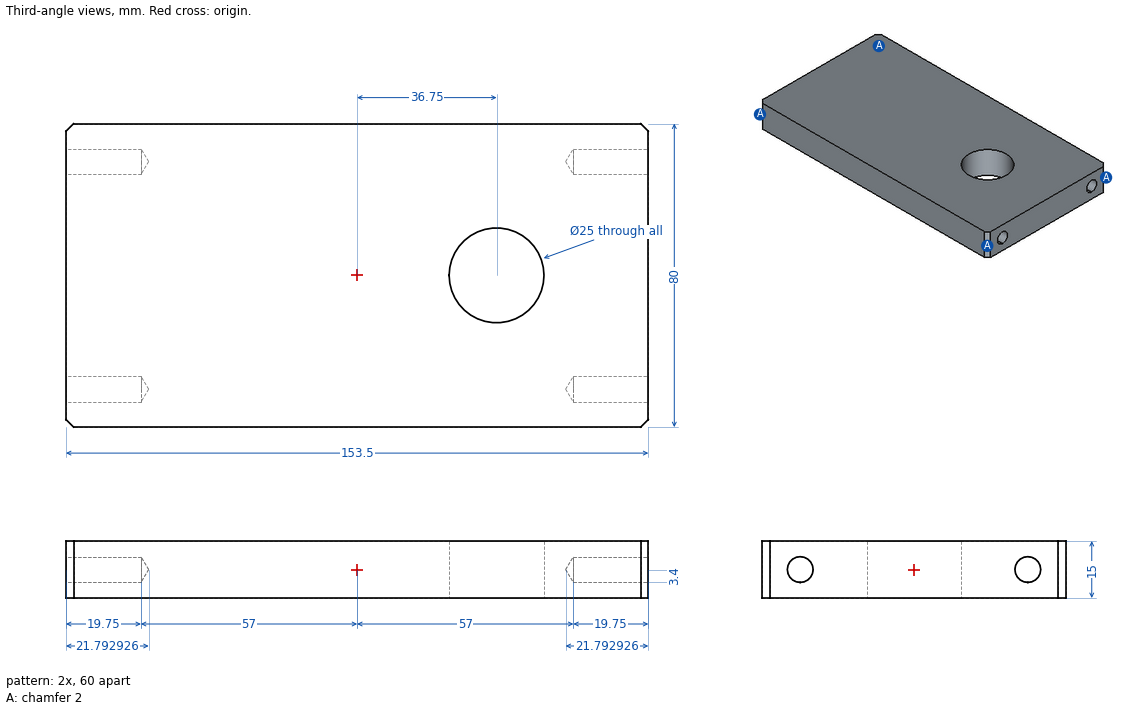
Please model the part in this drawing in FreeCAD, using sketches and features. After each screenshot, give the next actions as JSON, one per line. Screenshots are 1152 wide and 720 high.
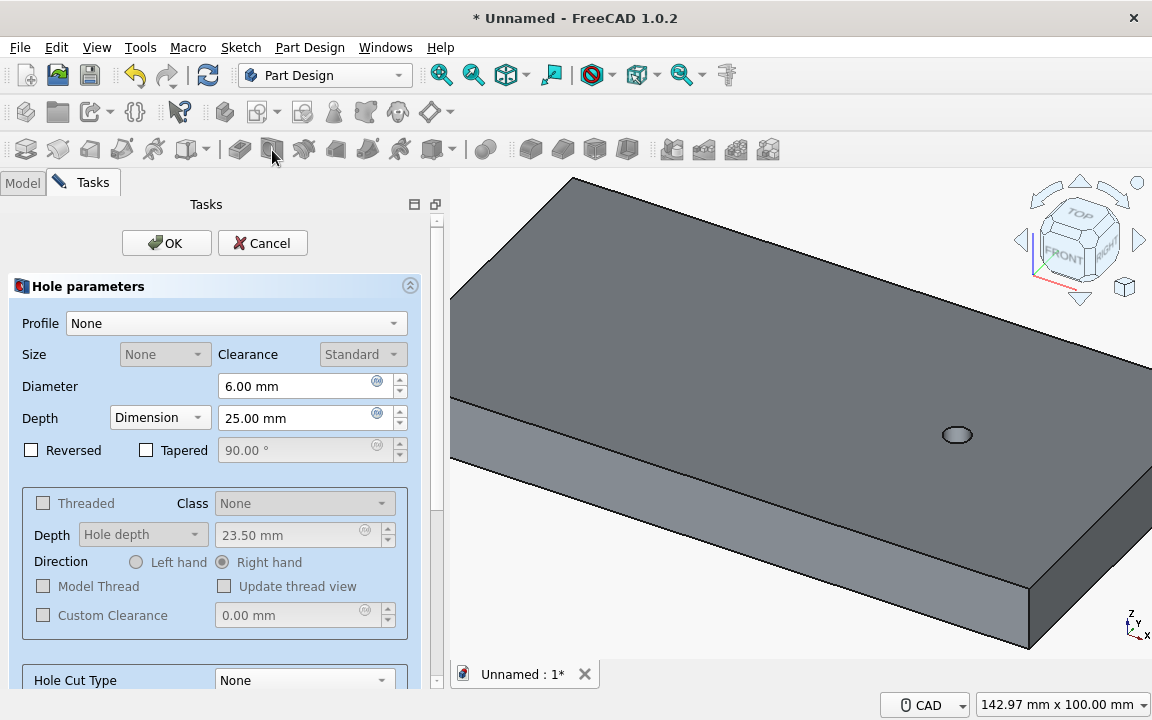
{"action": "triple_click", "coordinate": [305, 386]}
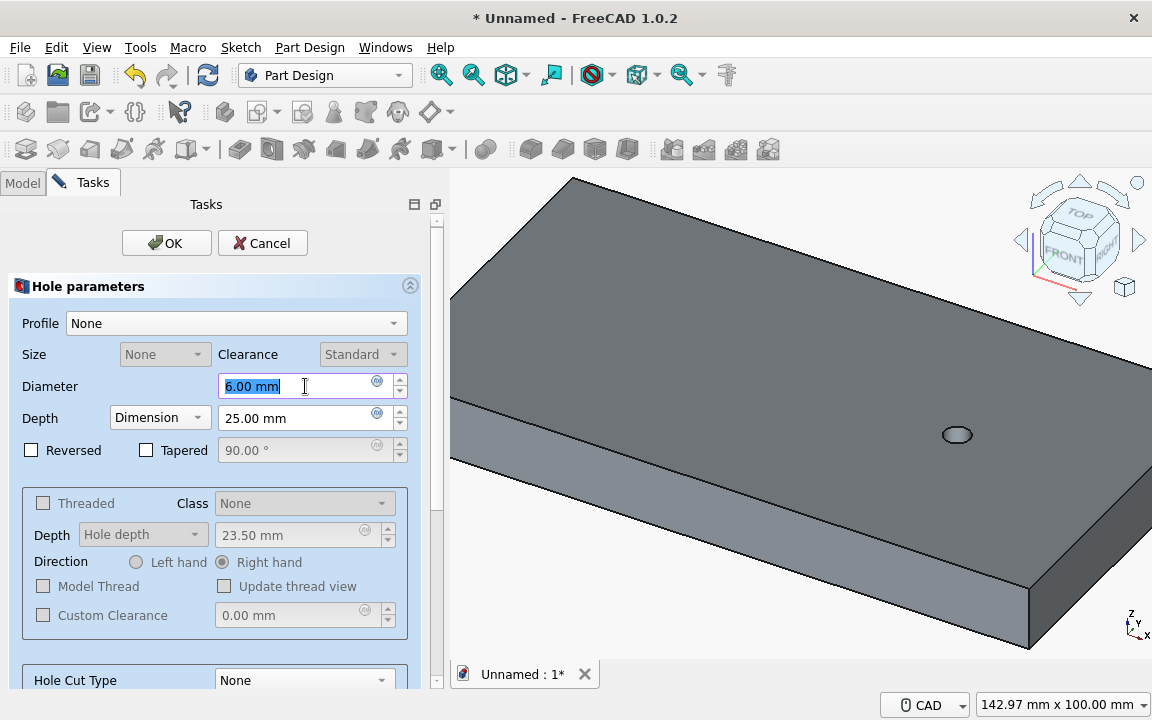
{"action": "type", "text": "25"}
{"action": "key", "text": "Tab"}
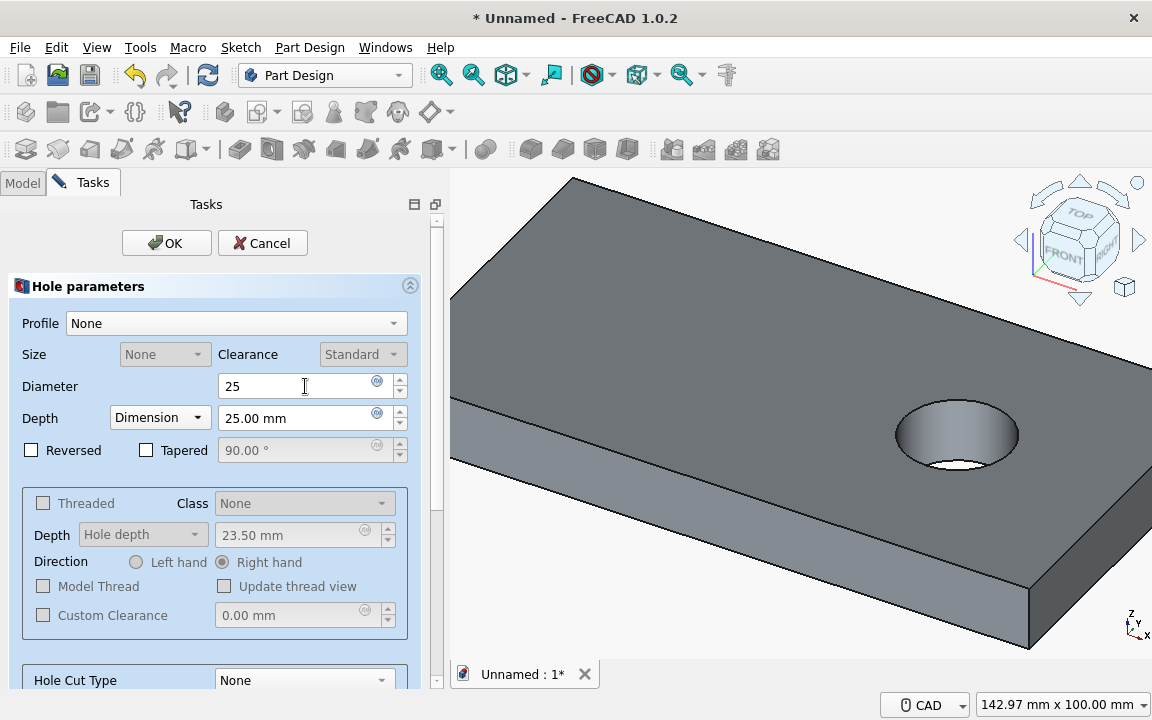
{"action": "left_click", "coordinate": [161, 418]}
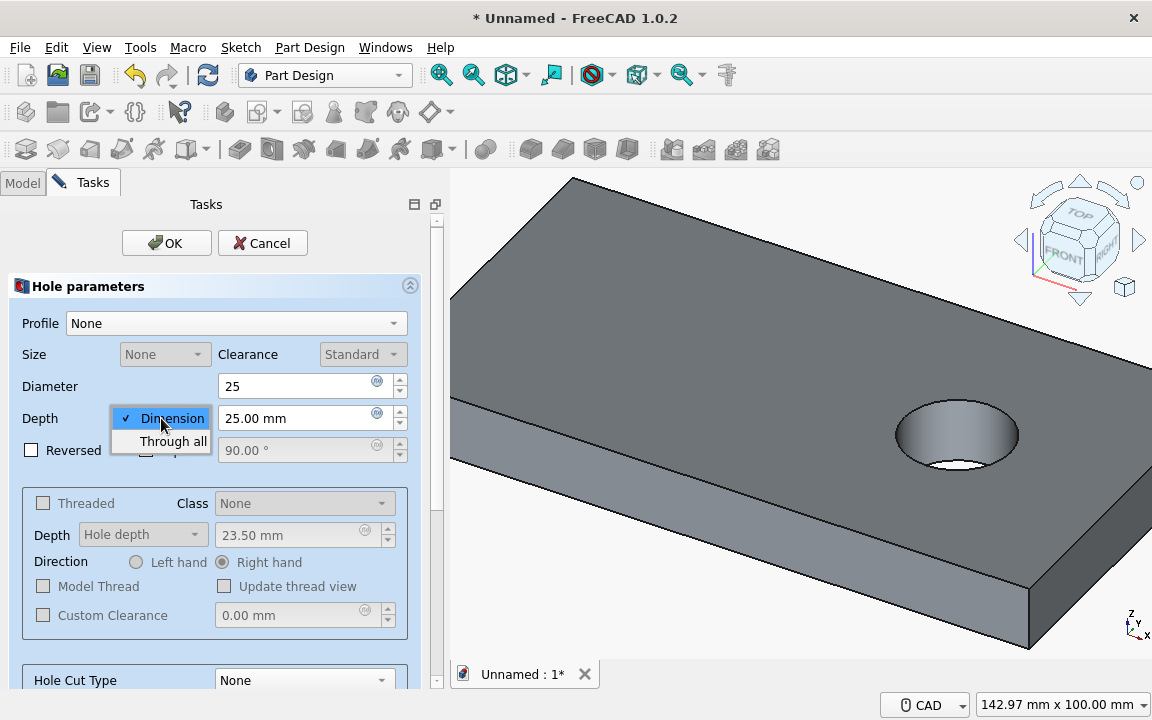
{"action": "left_click", "coordinate": [160, 442]}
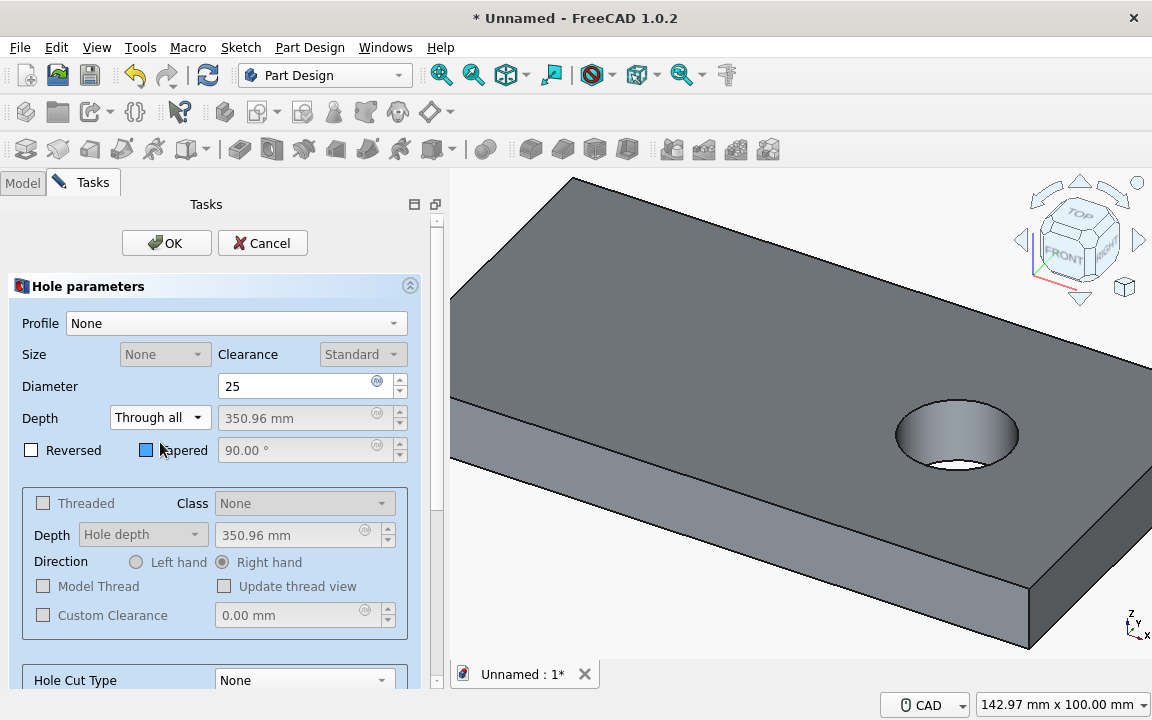
{"action": "left_click", "coordinate": [167, 243]}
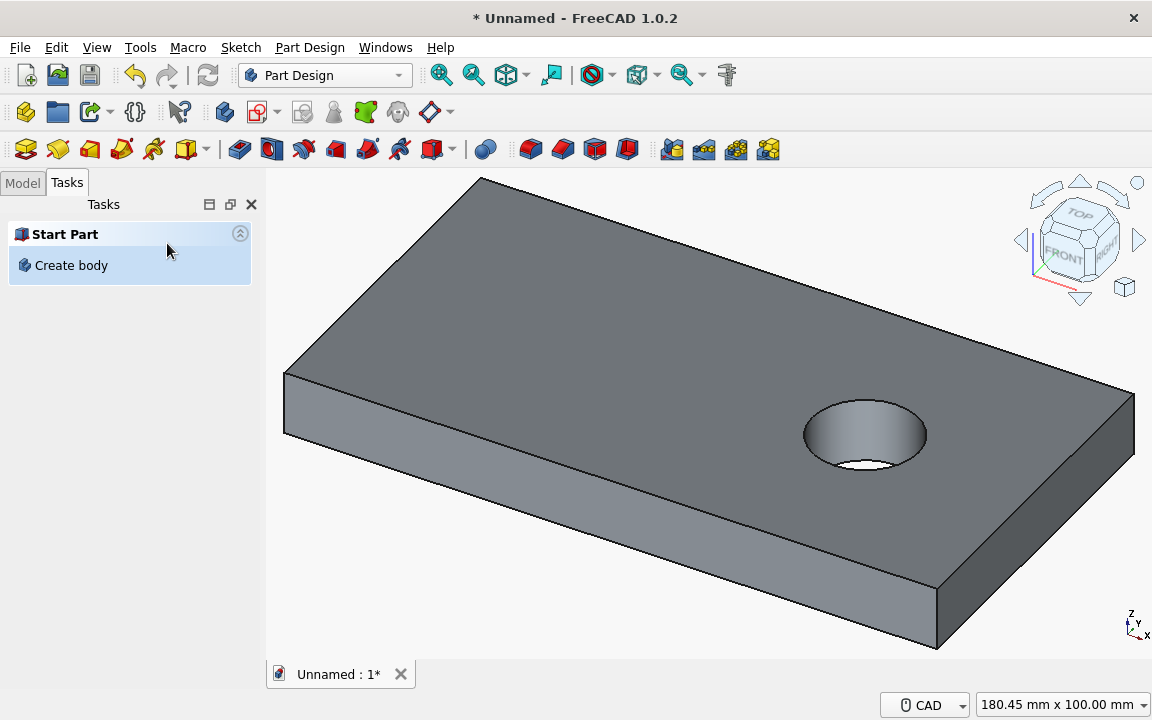
{"action": "left_click", "coordinate": [23, 182]}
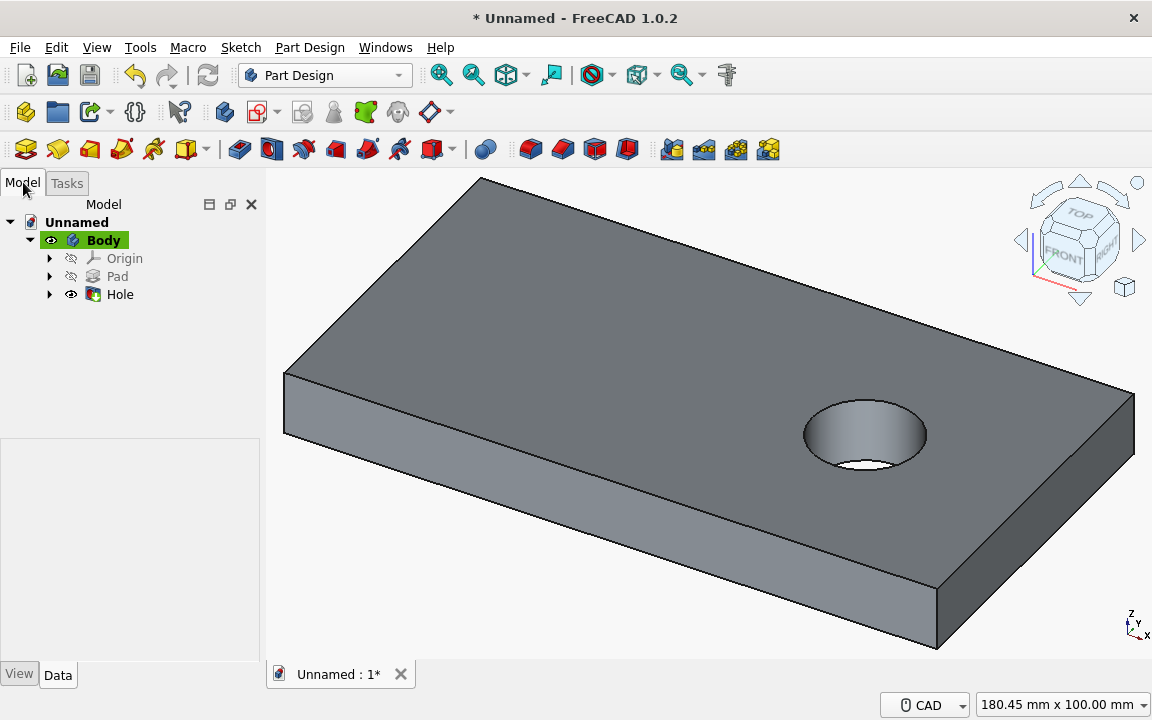
{"action": "left_click", "coordinate": [50, 258]}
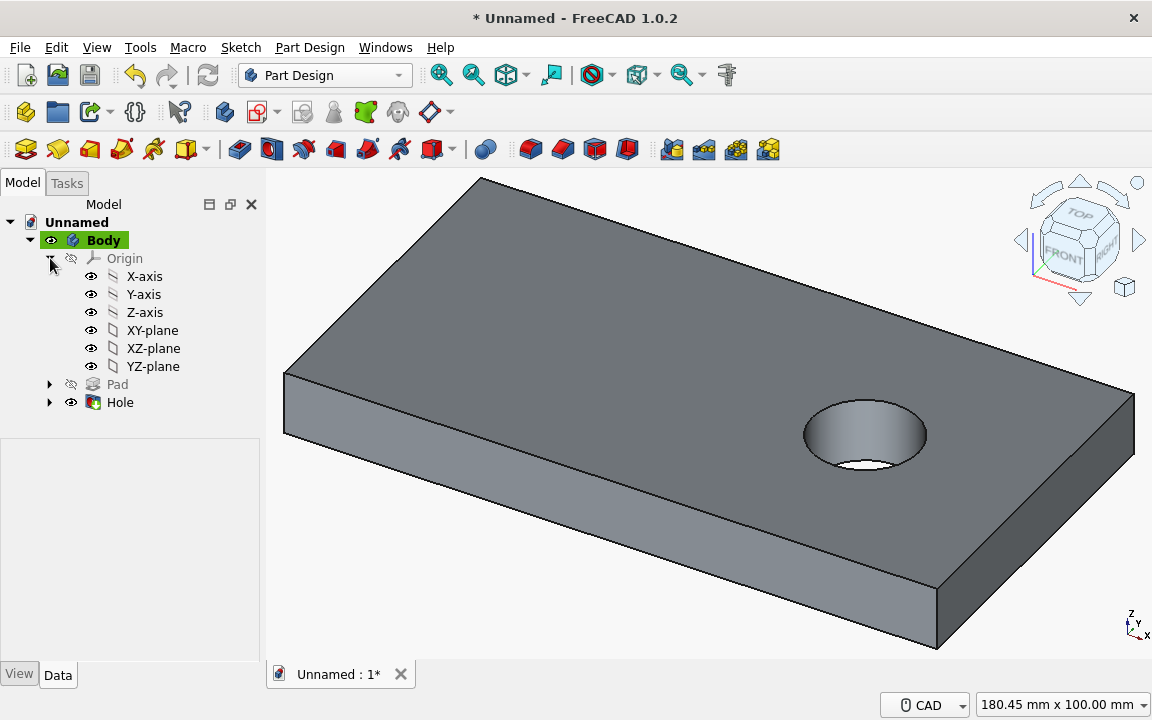
{"action": "left_click", "coordinate": [136, 348]}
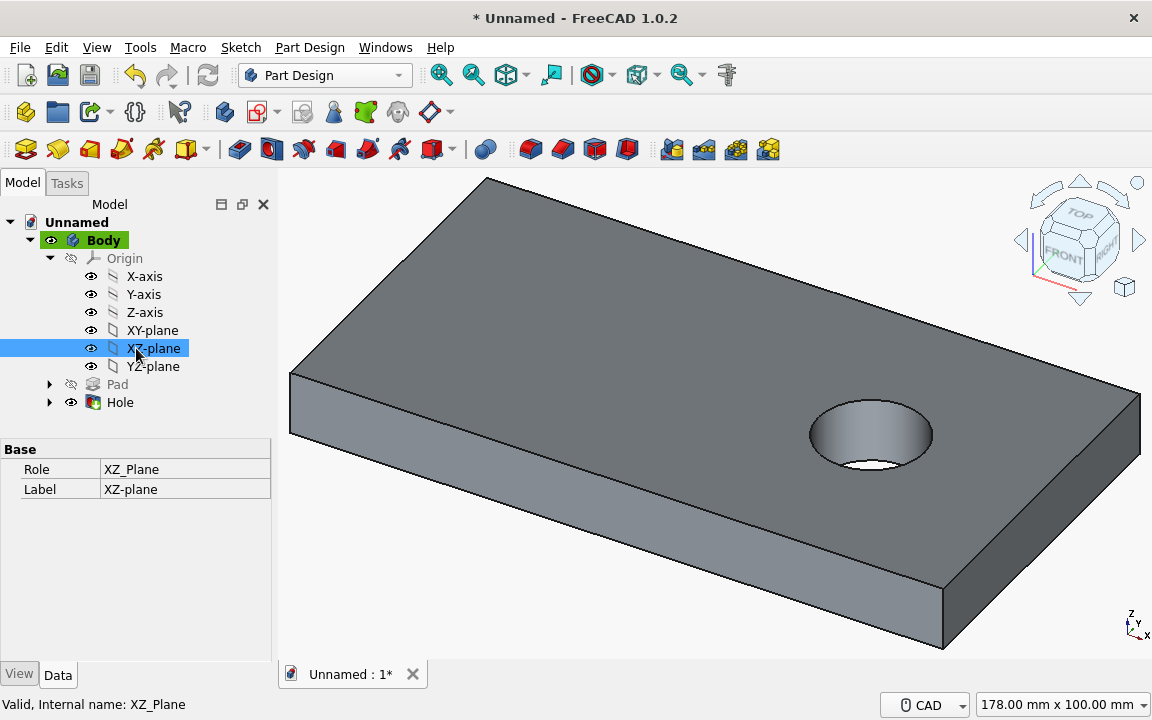
{"action": "left_click", "coordinate": [430, 112]}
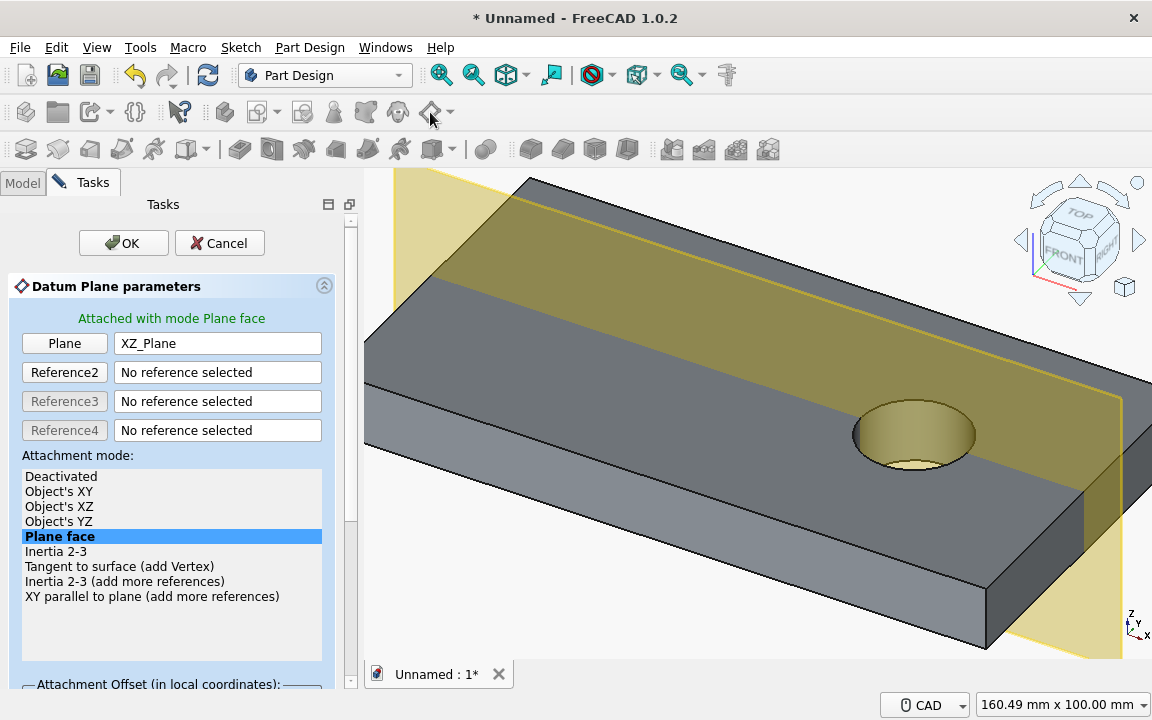
{"action": "scroll", "coordinate": [351, 451], "scroll_direction": "down", "scroll_amount": 3}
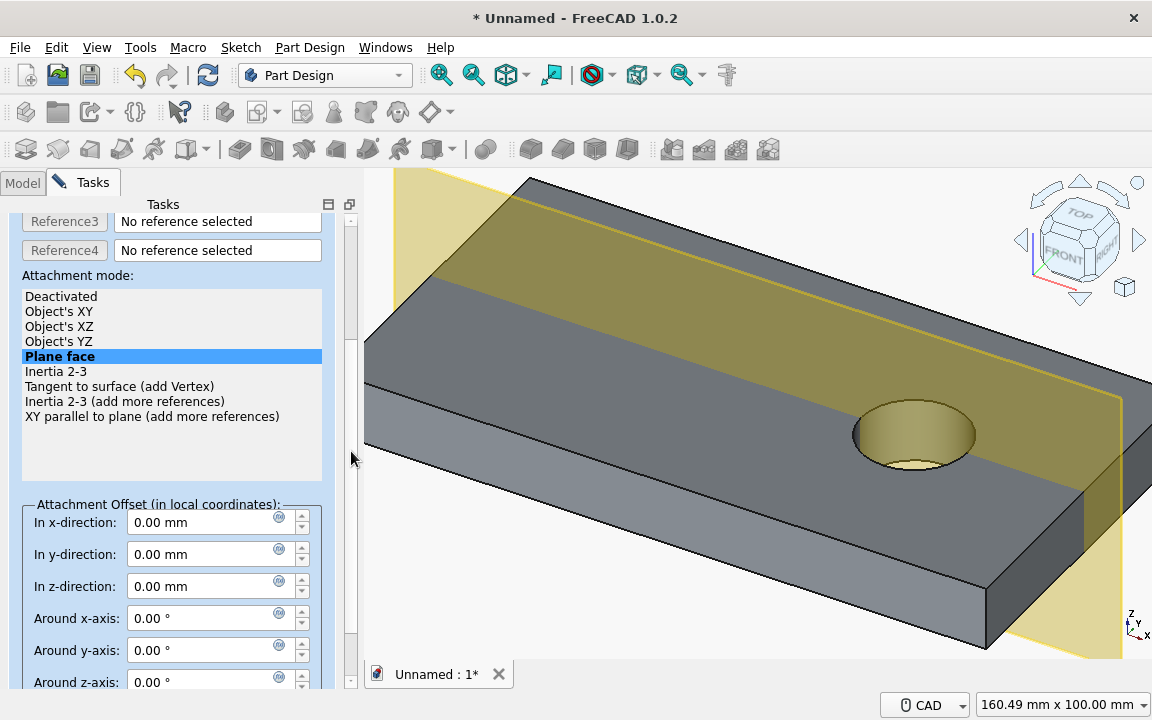
{"action": "triple_click", "coordinate": [210, 586]}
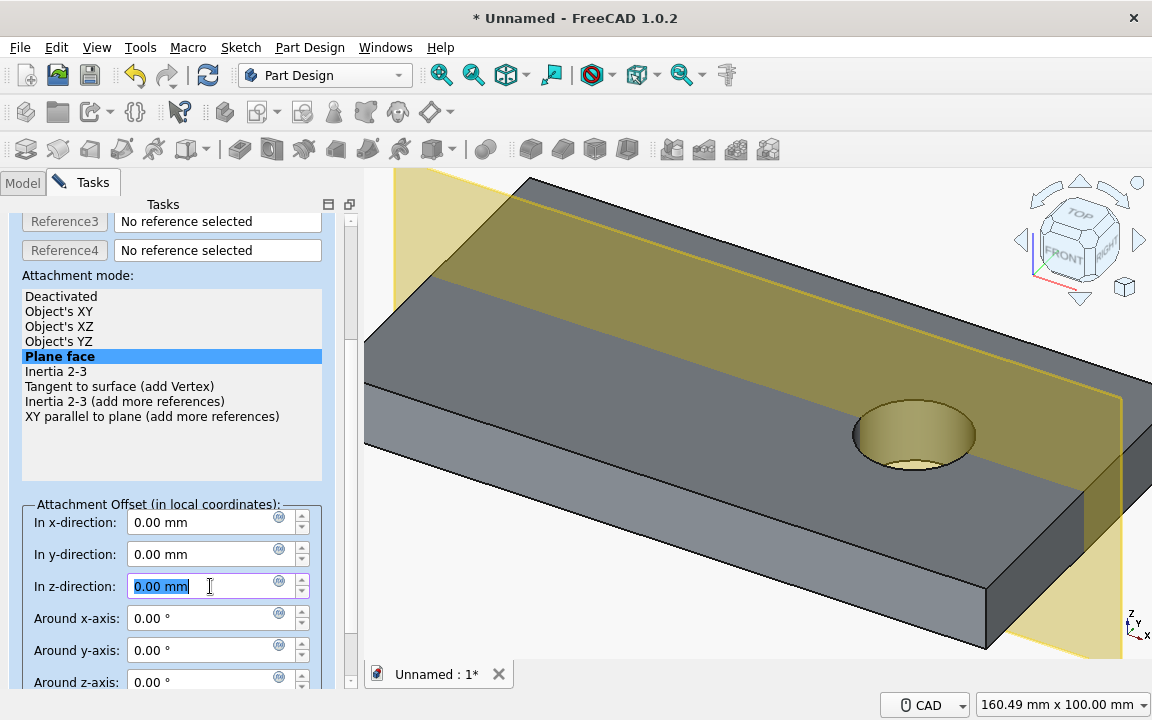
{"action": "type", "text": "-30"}
{"action": "key", "text": "Tab"}